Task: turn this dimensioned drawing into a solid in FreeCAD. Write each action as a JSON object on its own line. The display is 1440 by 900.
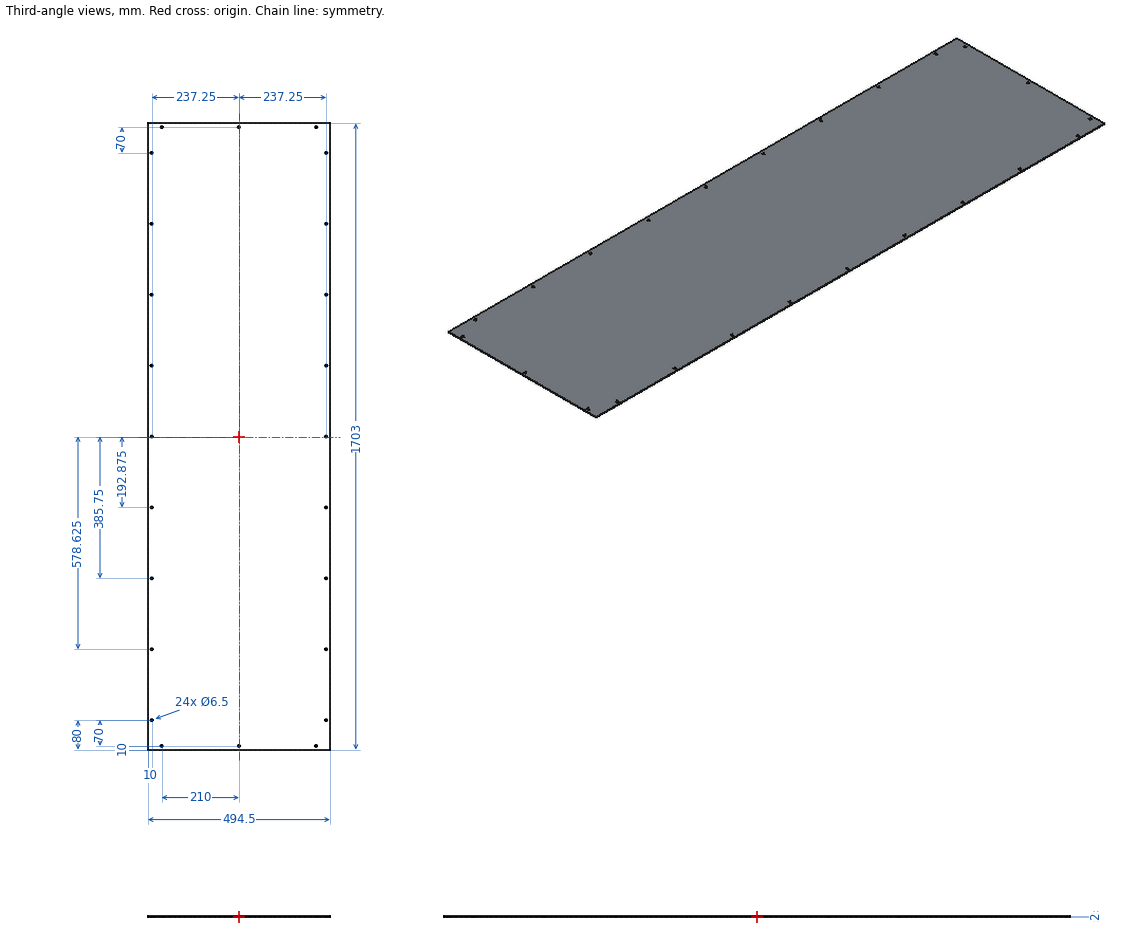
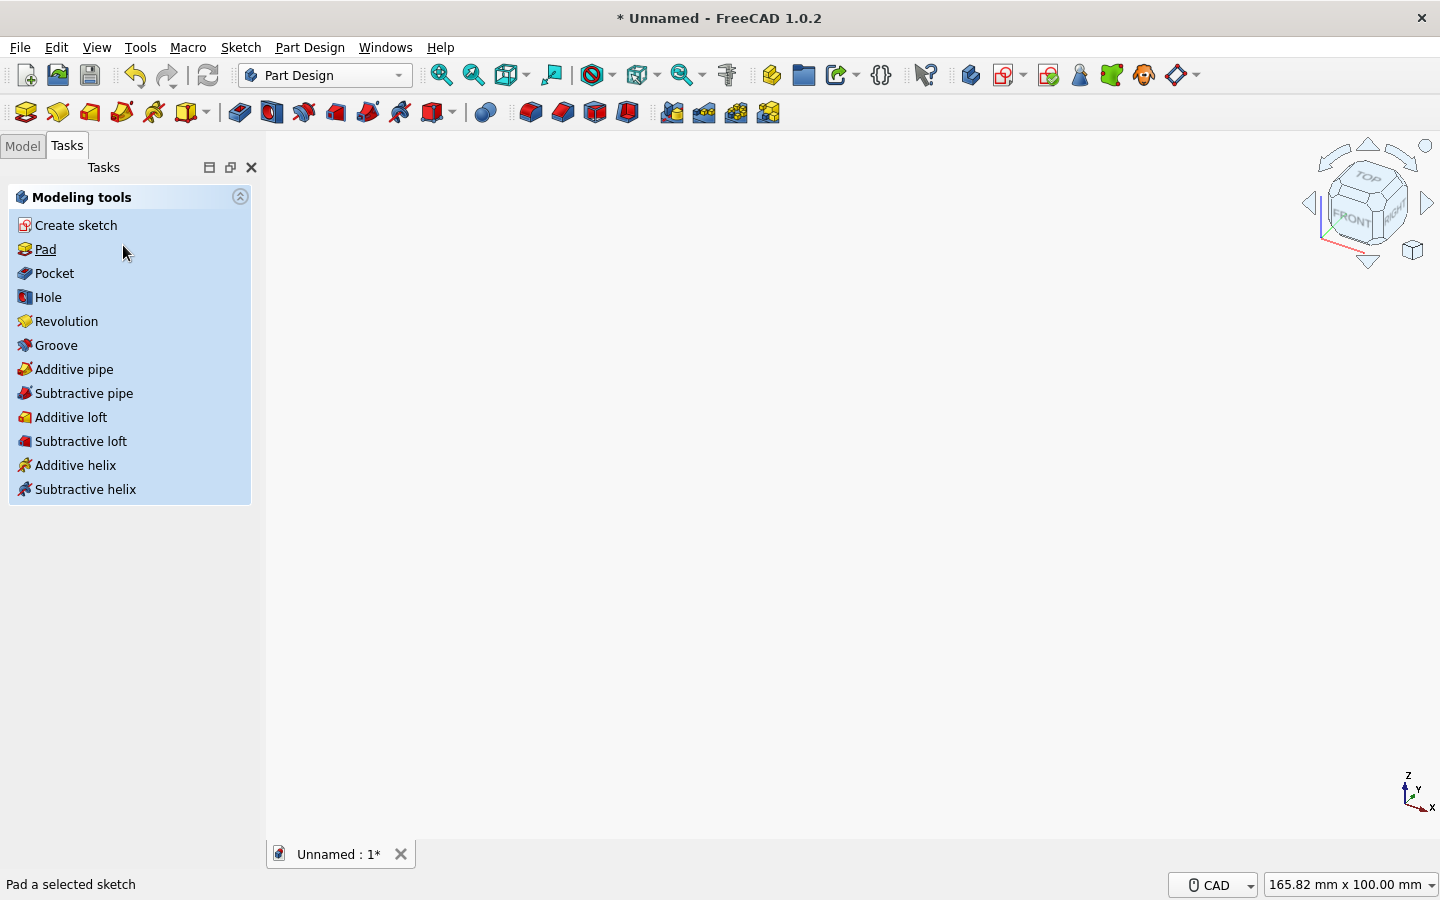
{"action": "left_click", "coordinate": [26, 112]}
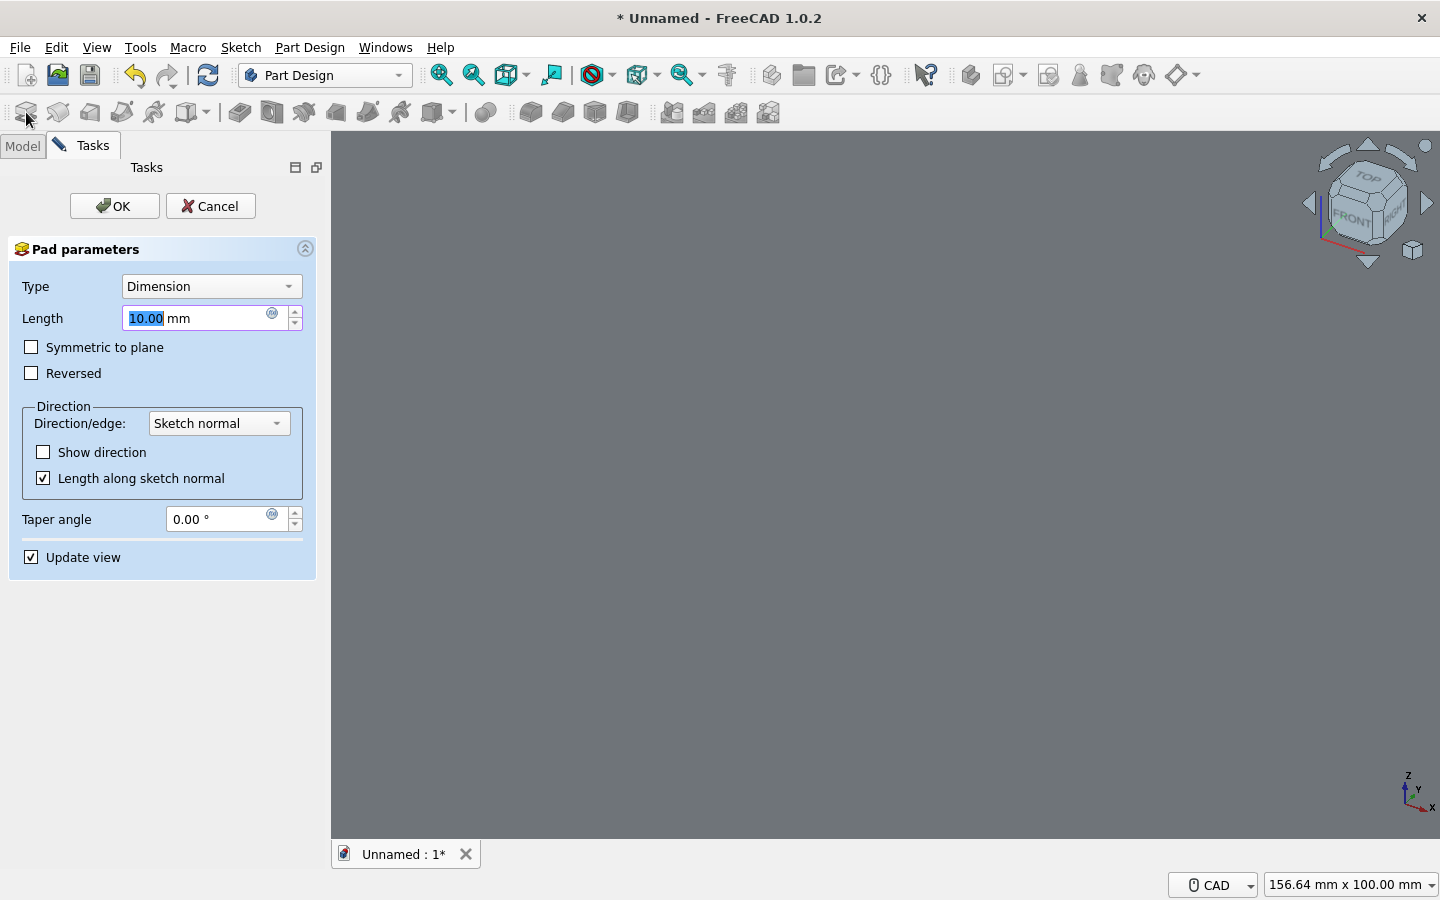
{"action": "type", "text": "2"}
{"action": "key", "text": "Tab"}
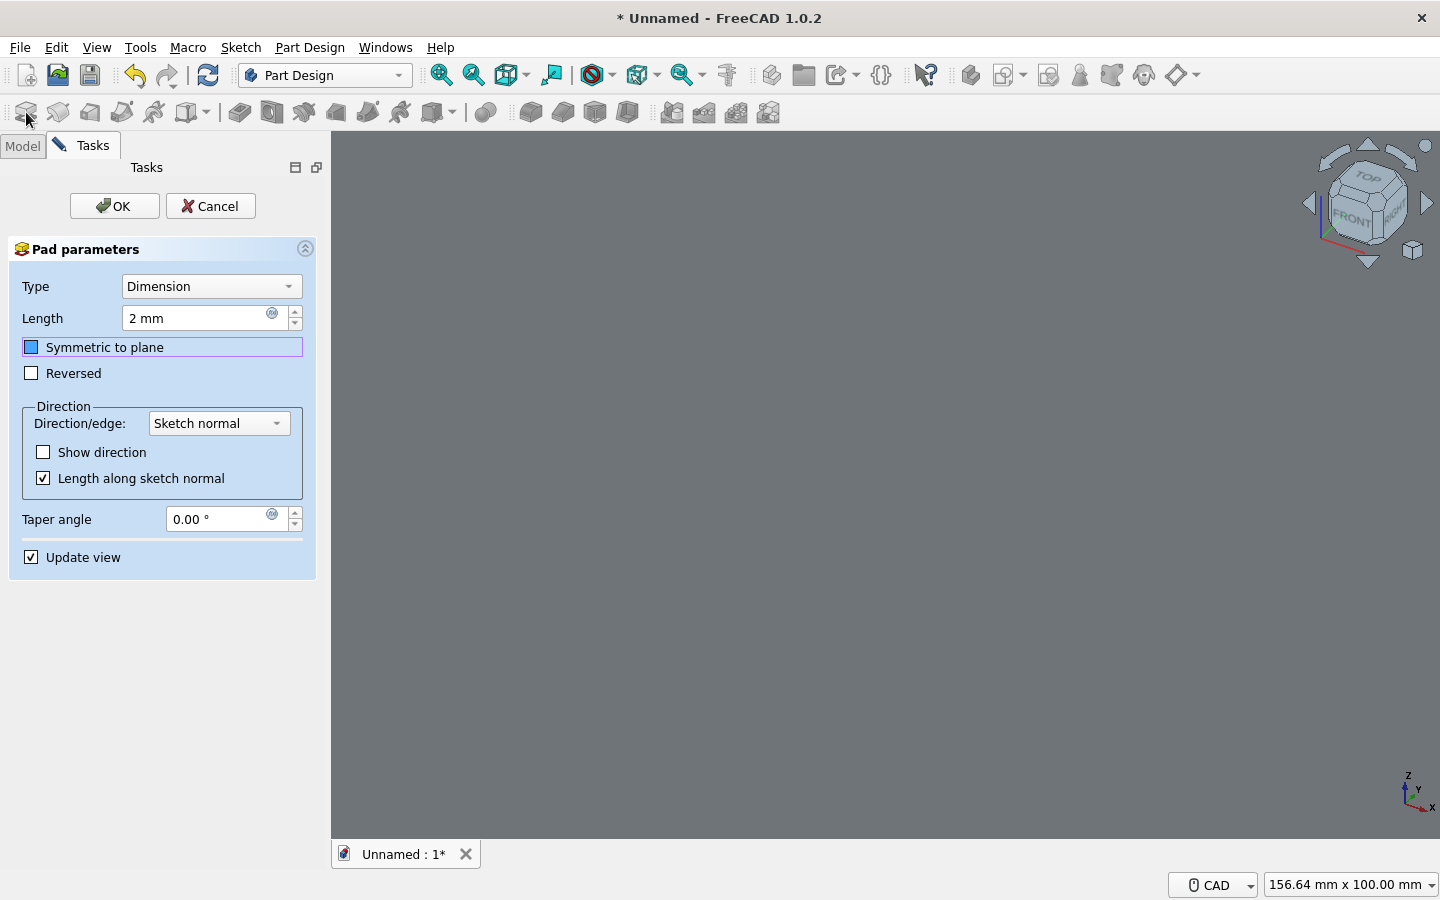
{"action": "left_click", "coordinate": [115, 206]}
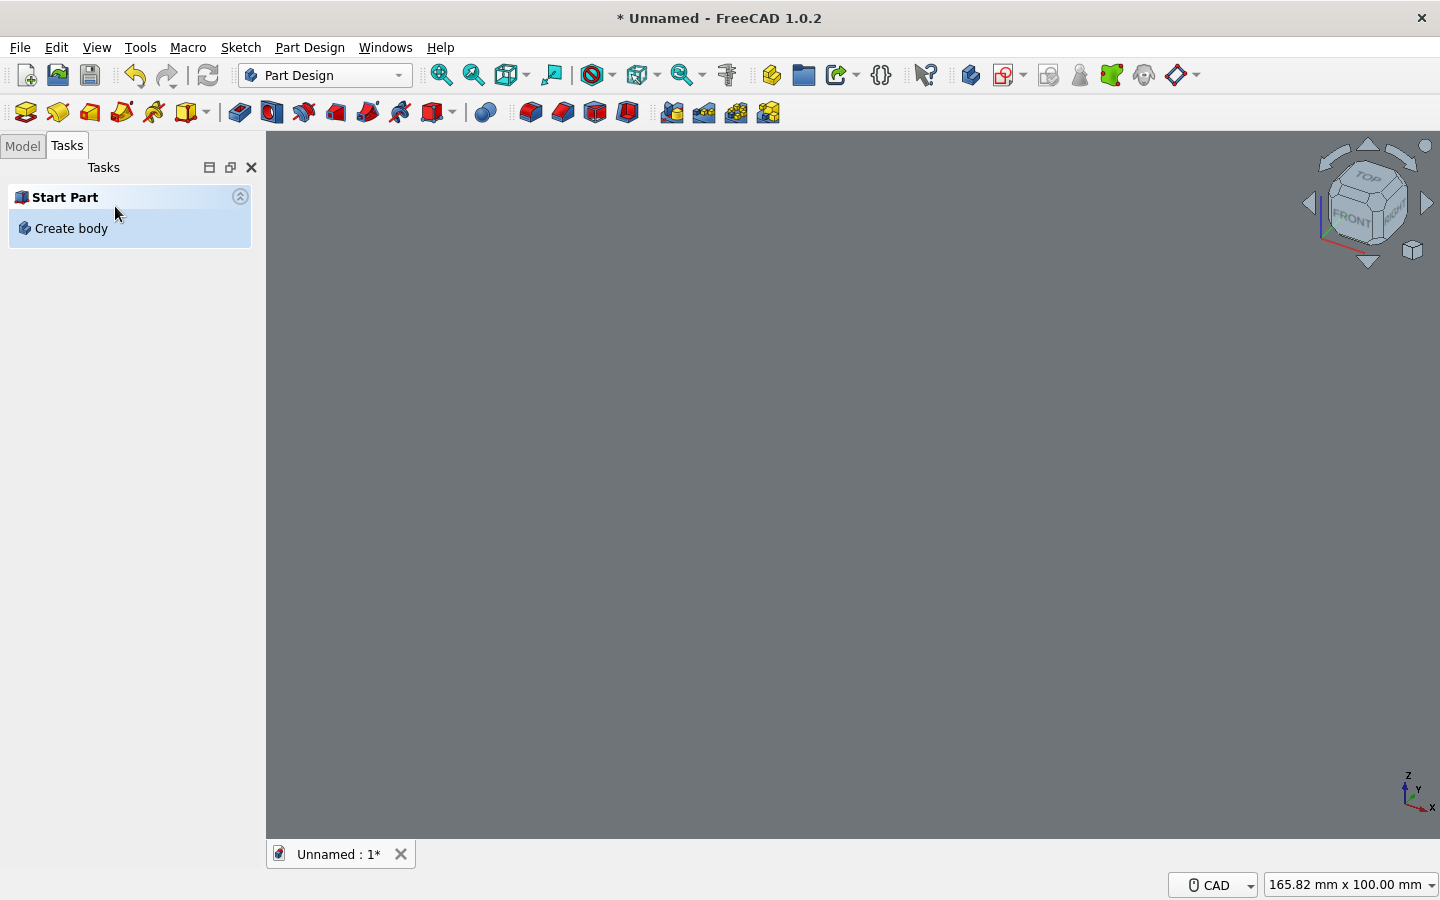
{"action": "key", "text": "0"}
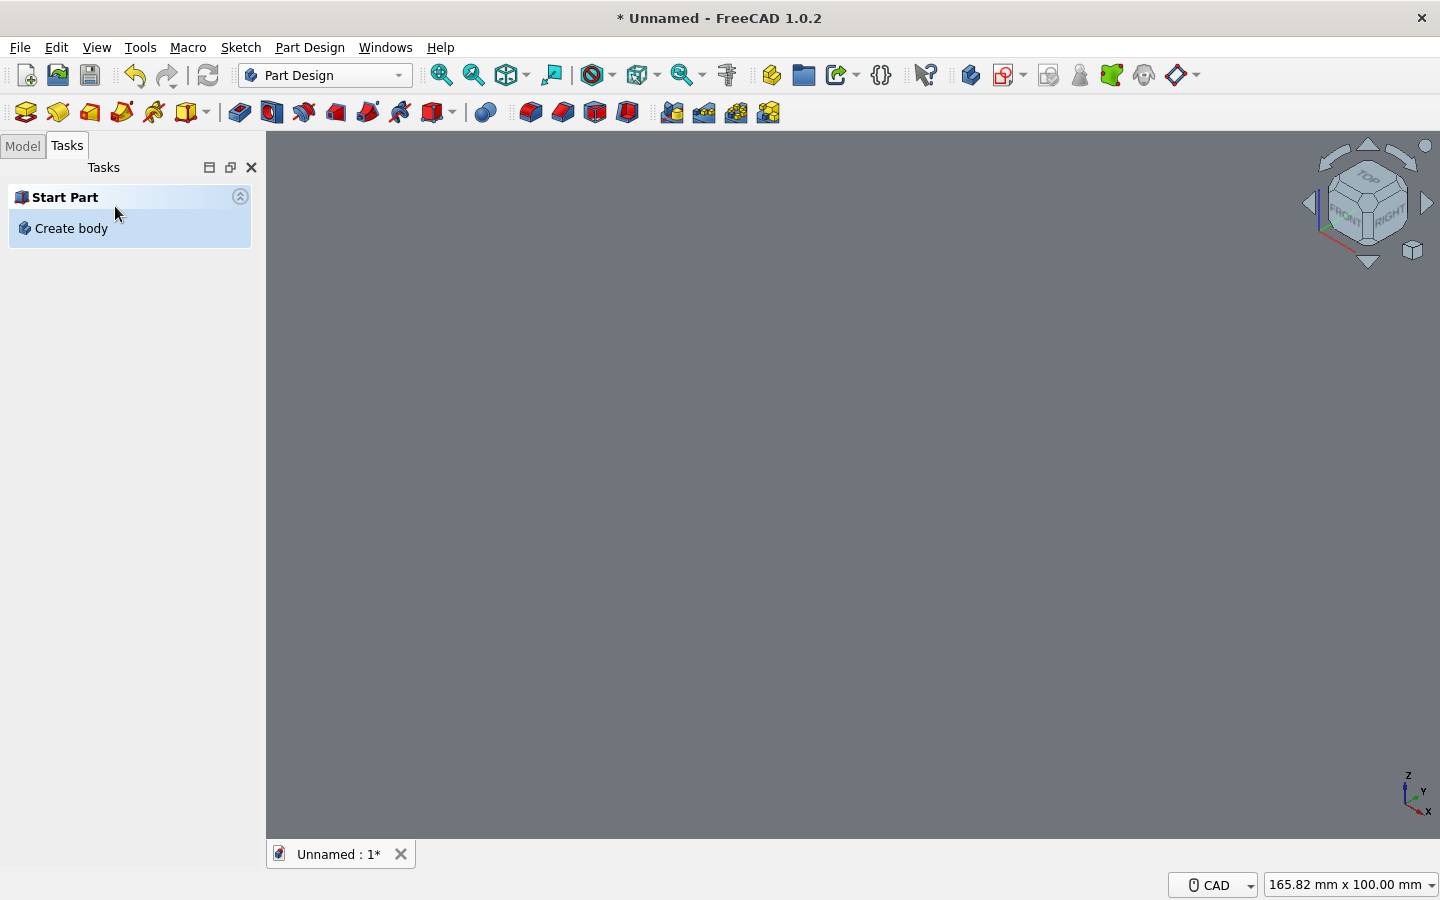
{"action": "left_click", "coordinate": [442, 76]}